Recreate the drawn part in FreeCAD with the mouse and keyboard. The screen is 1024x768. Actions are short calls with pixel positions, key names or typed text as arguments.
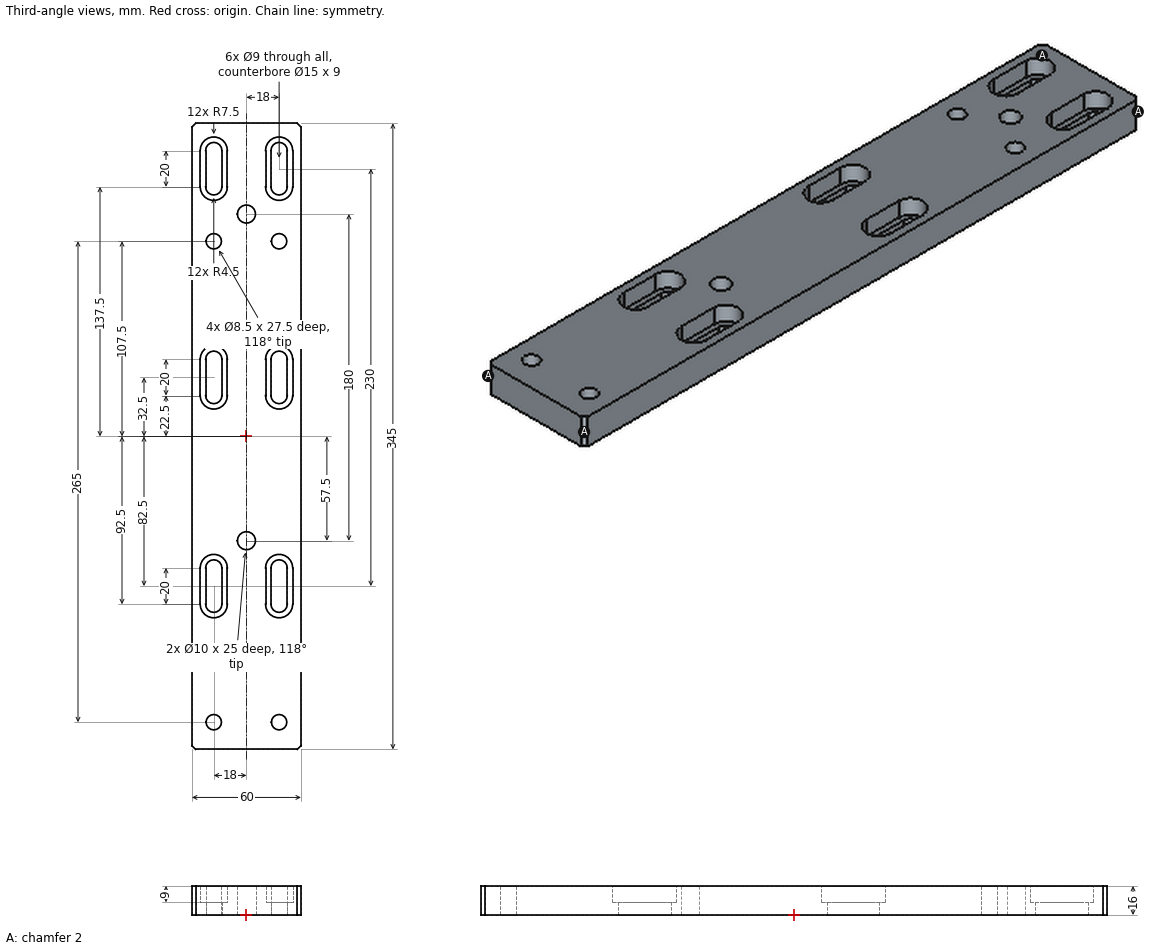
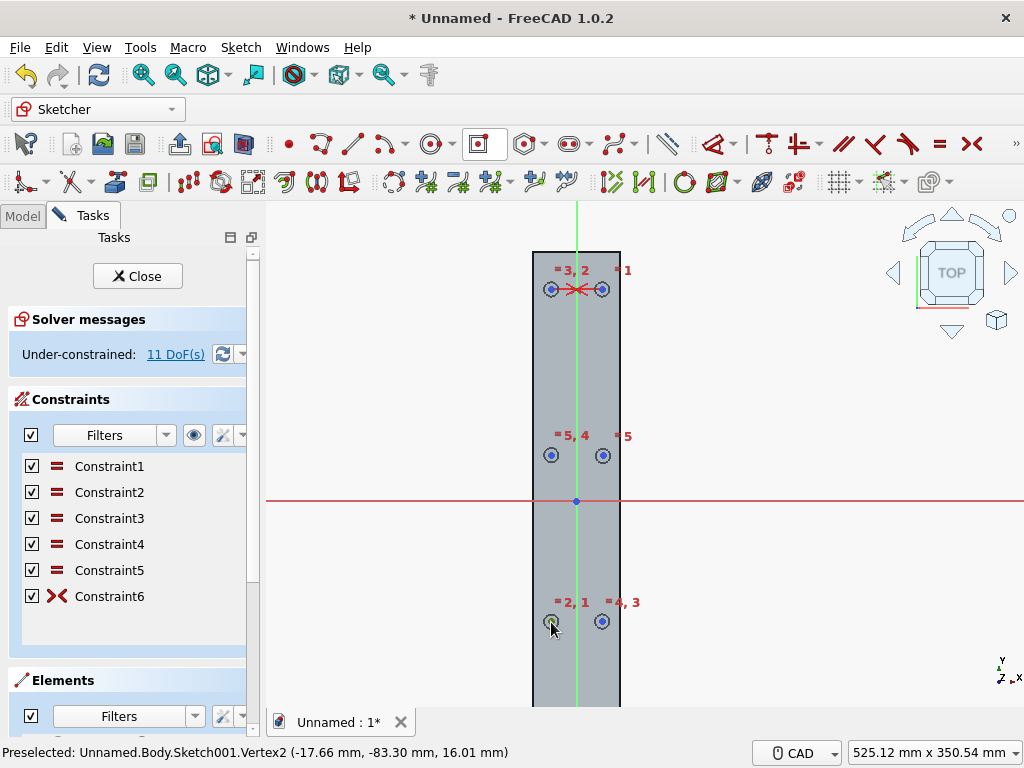
click(602, 622)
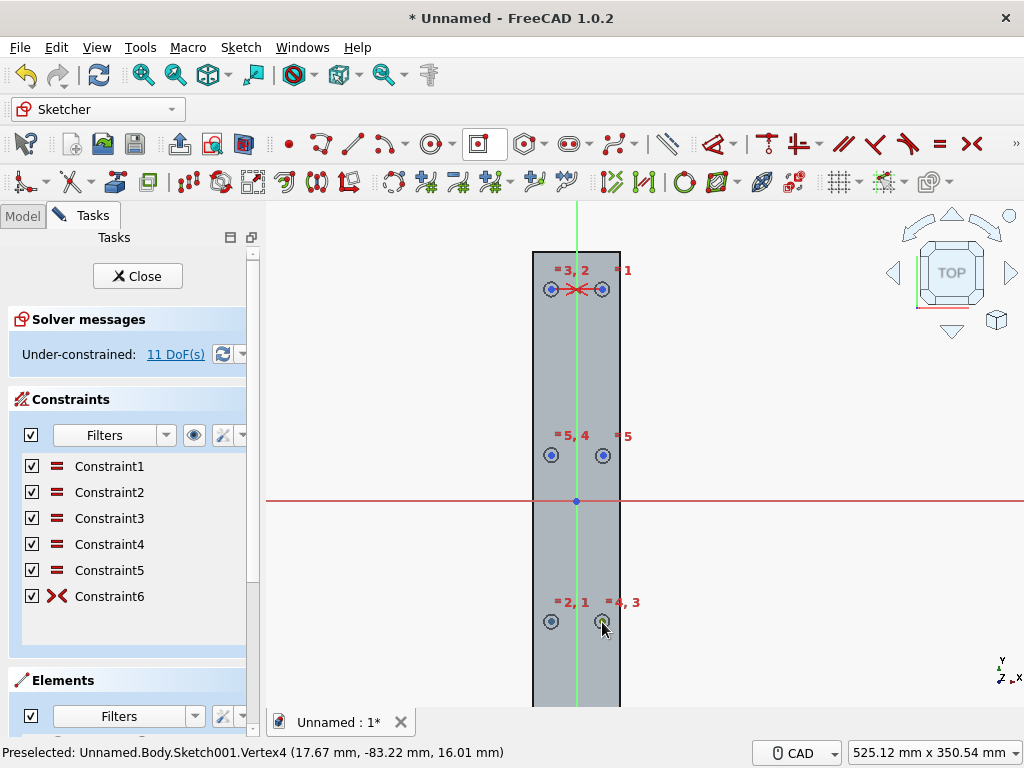
click(577, 583)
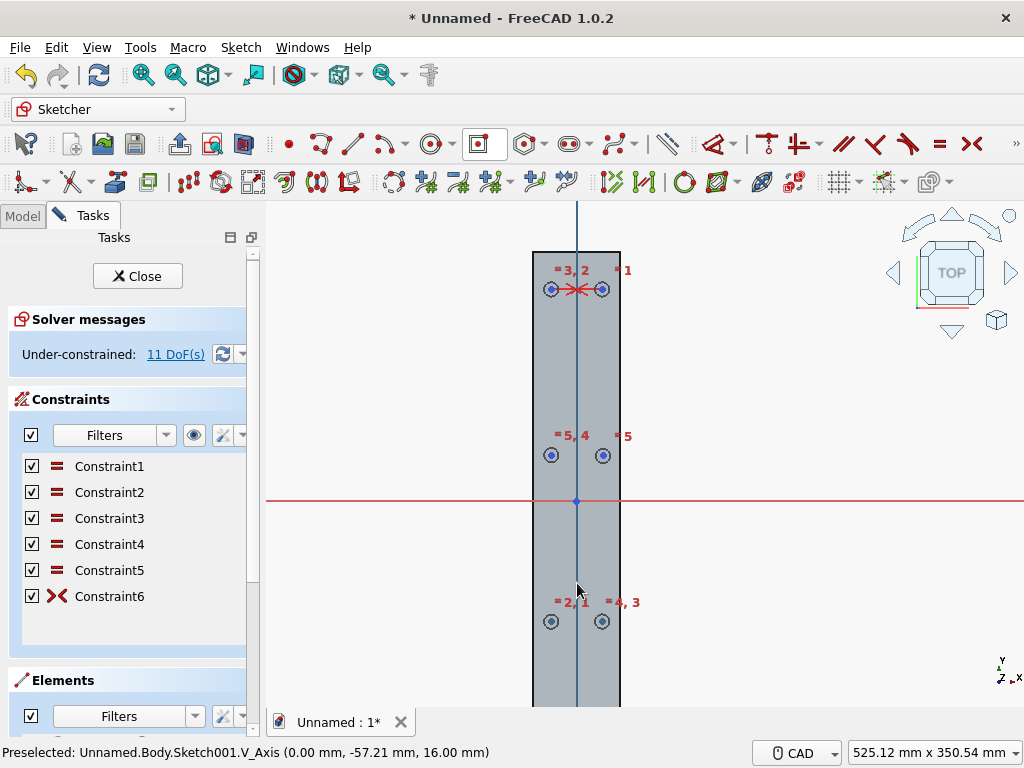
click(972, 144)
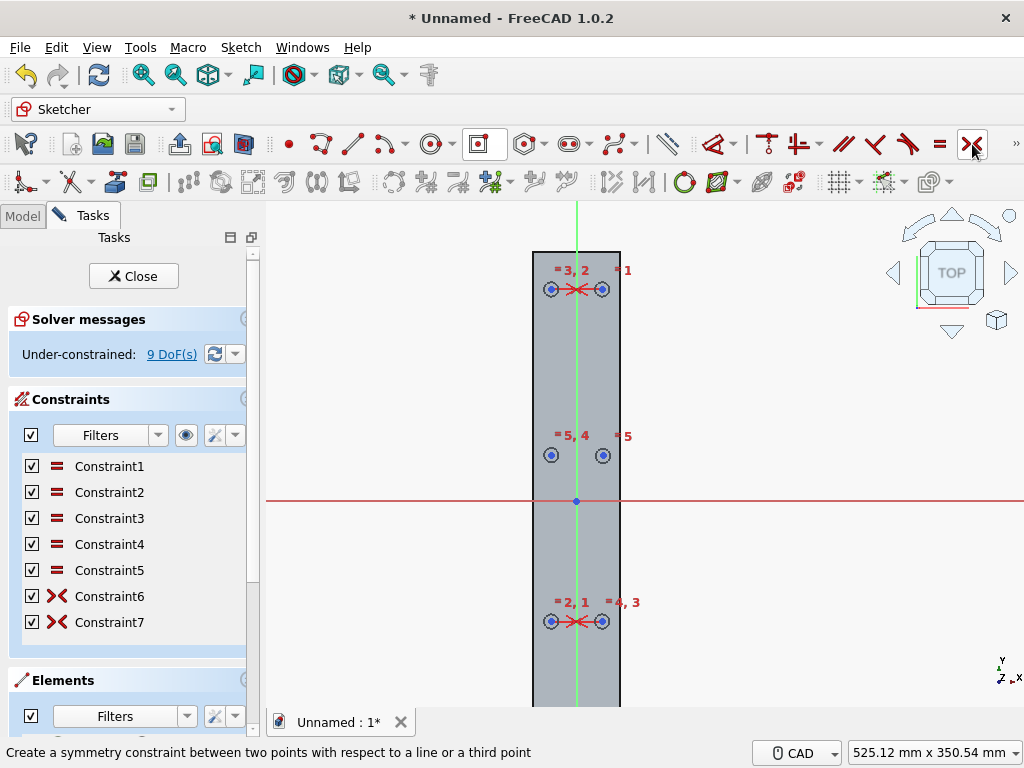
click(551, 455)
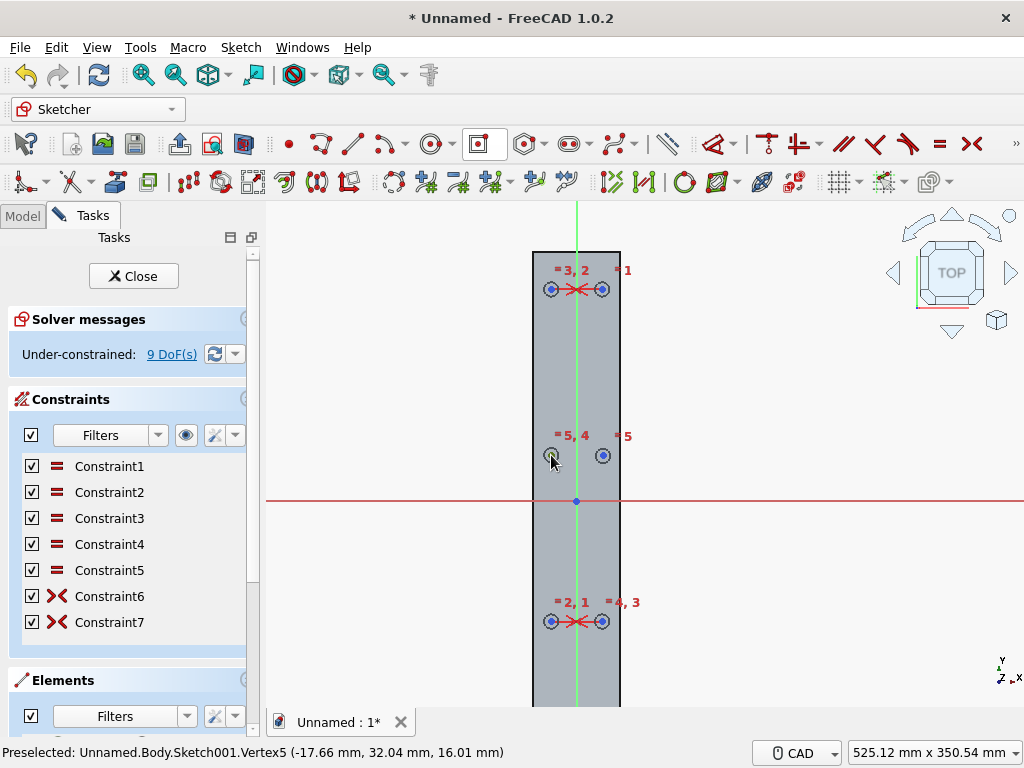
click(603, 456)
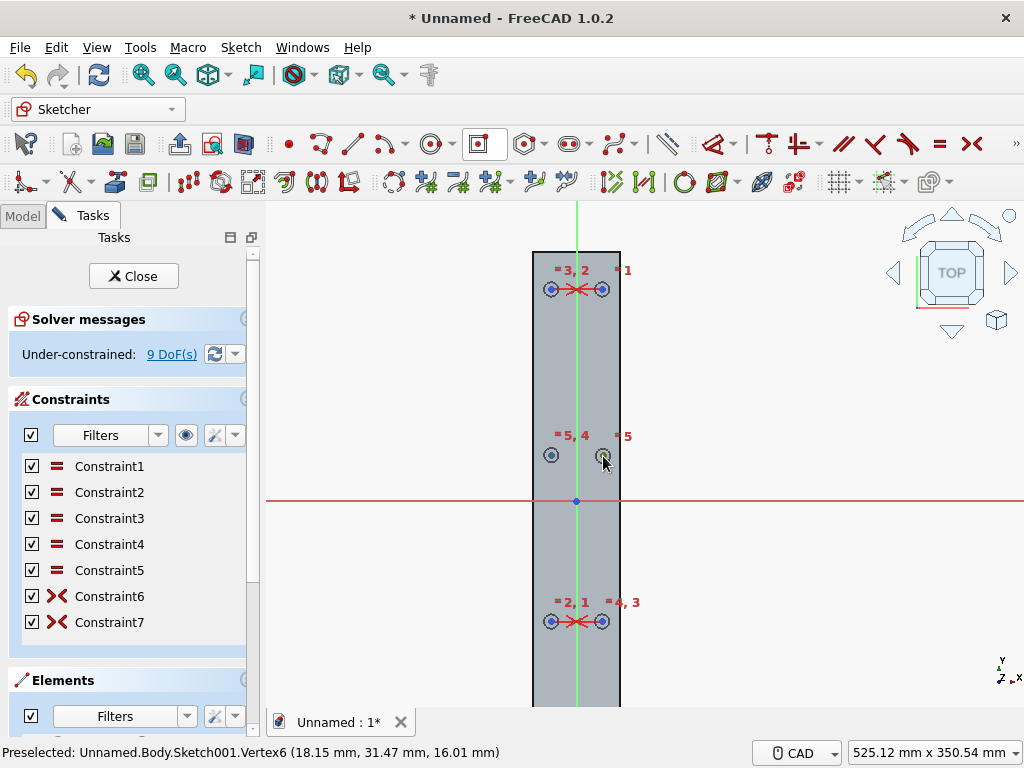
click(577, 583)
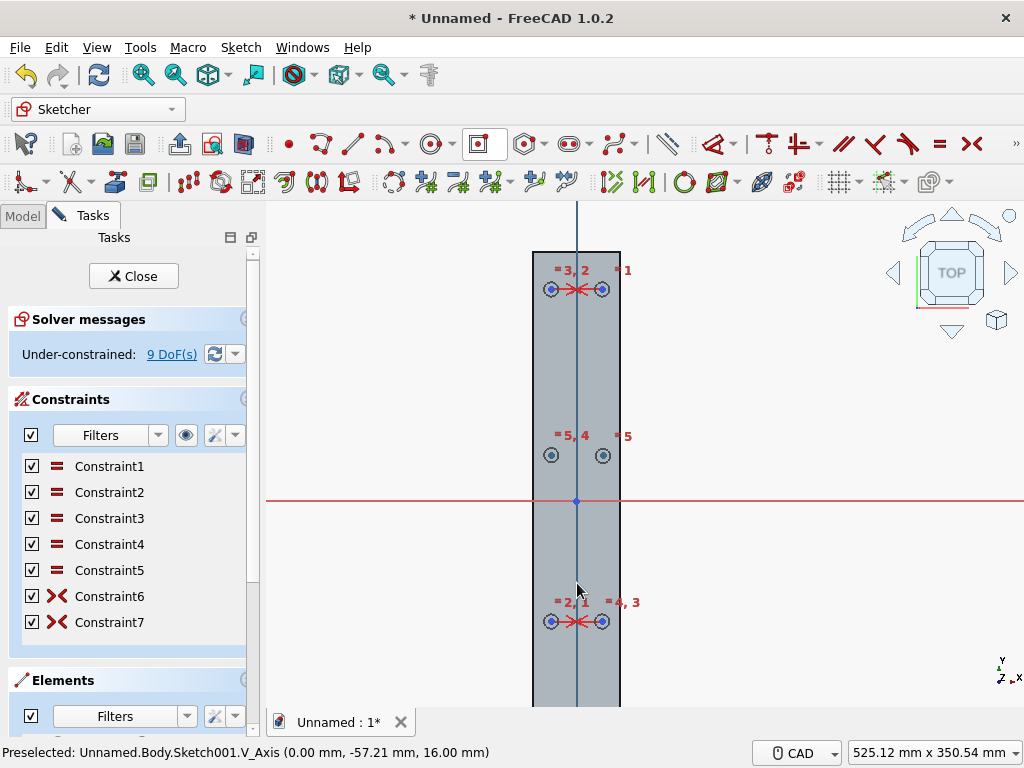
key(s)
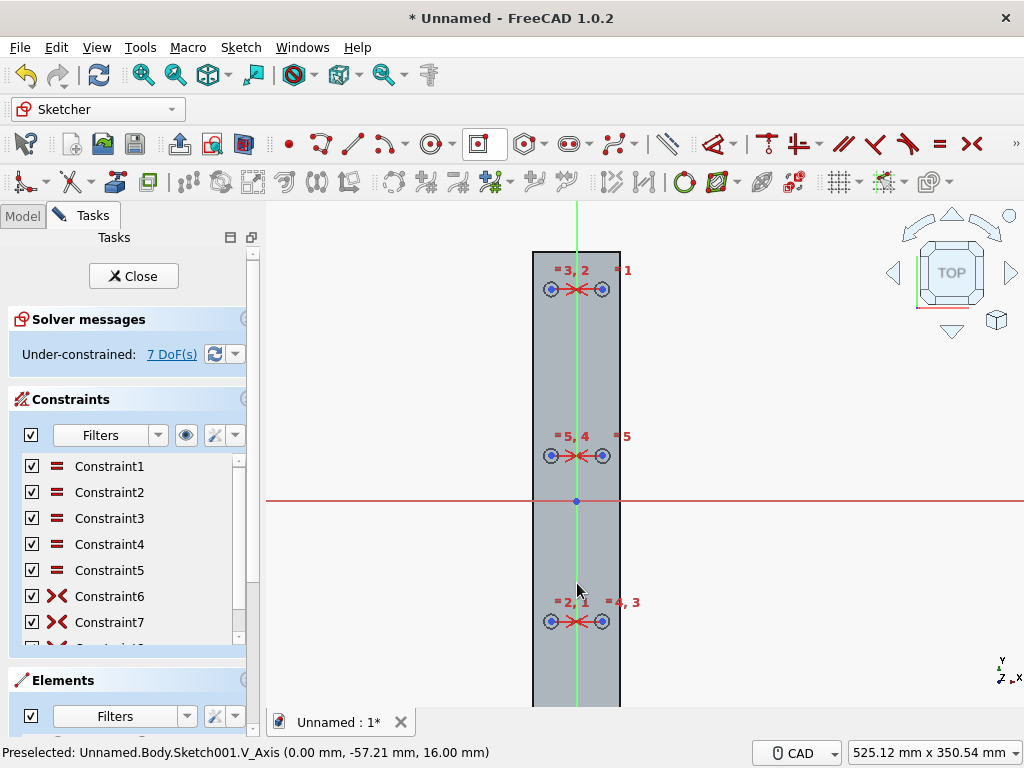
key(d)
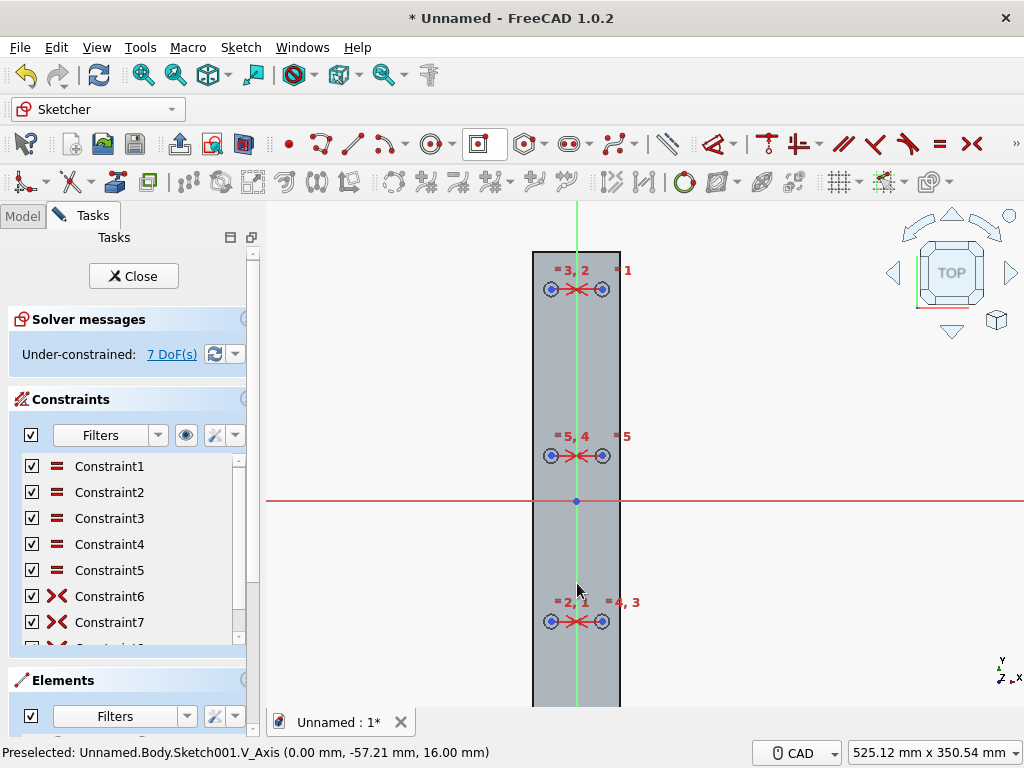
scroll(602, 282, up, 6)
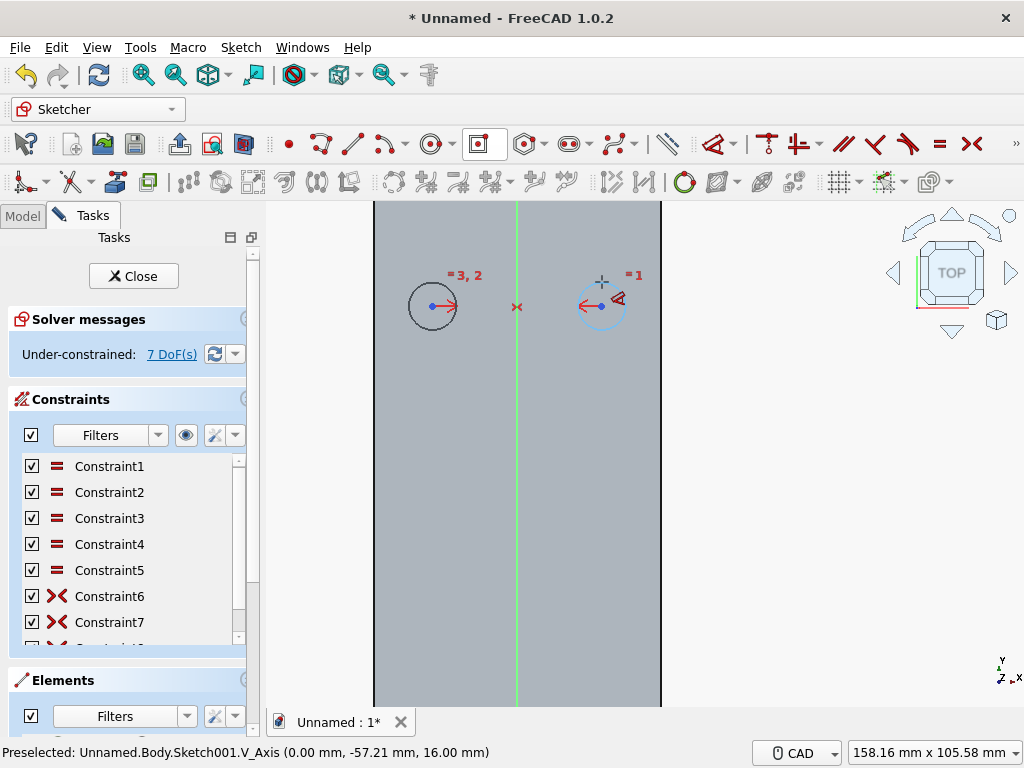
click(603, 283)
click(604, 251)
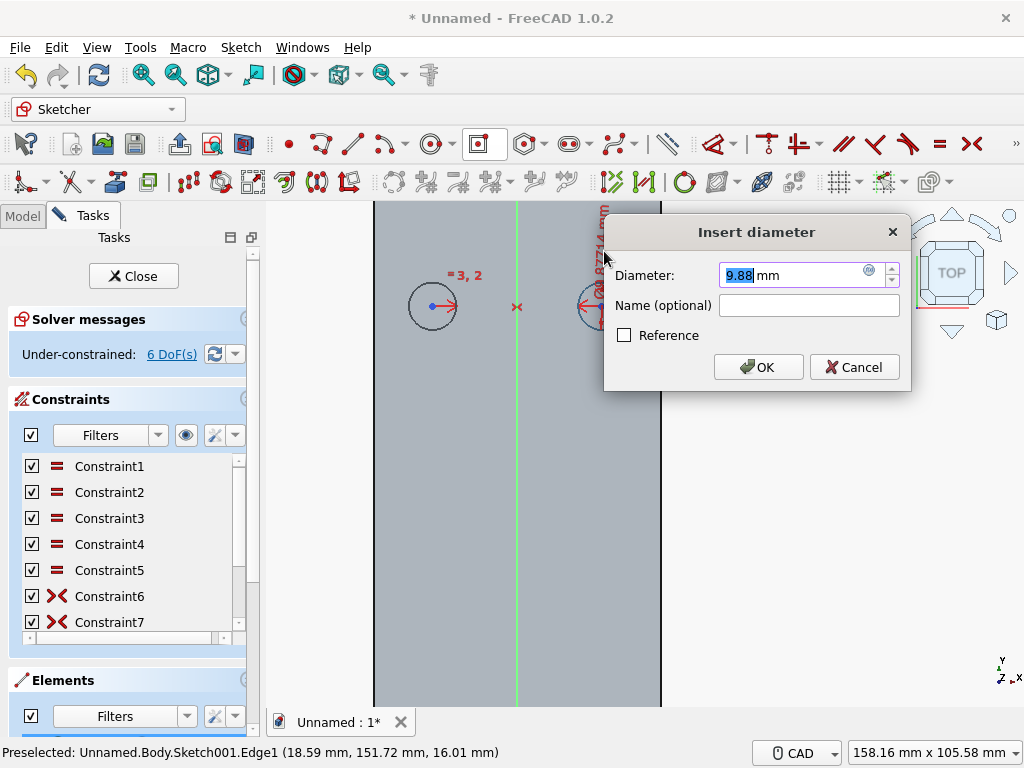
text(9)
key(Return)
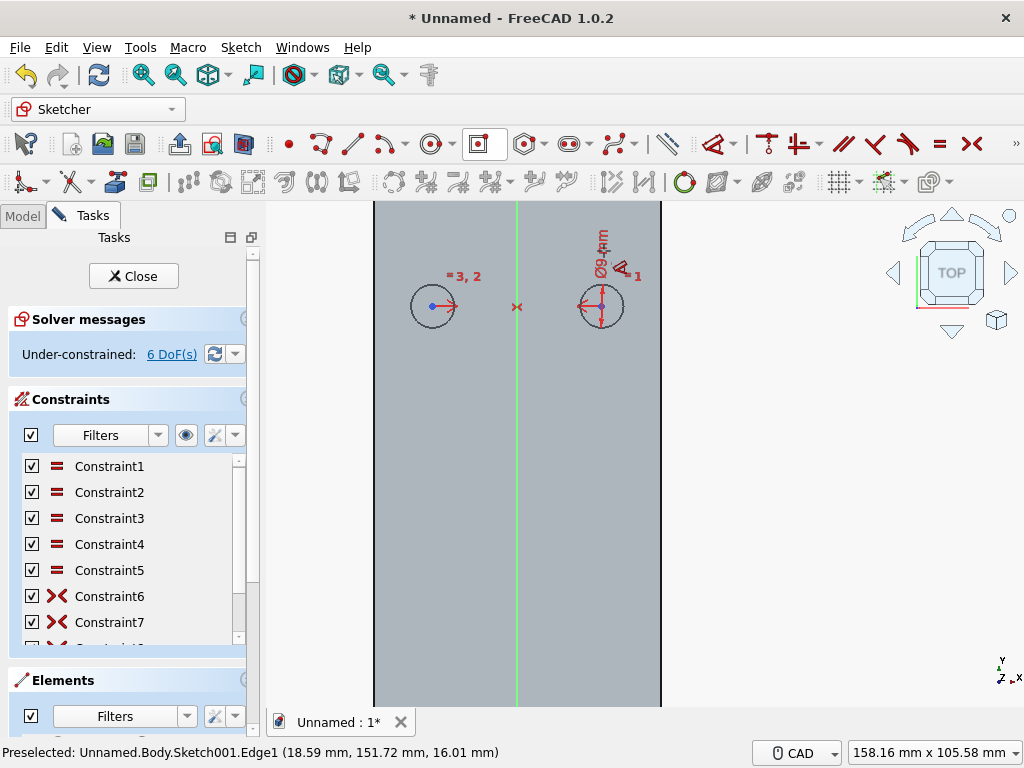
click(602, 306)
click(560, 272)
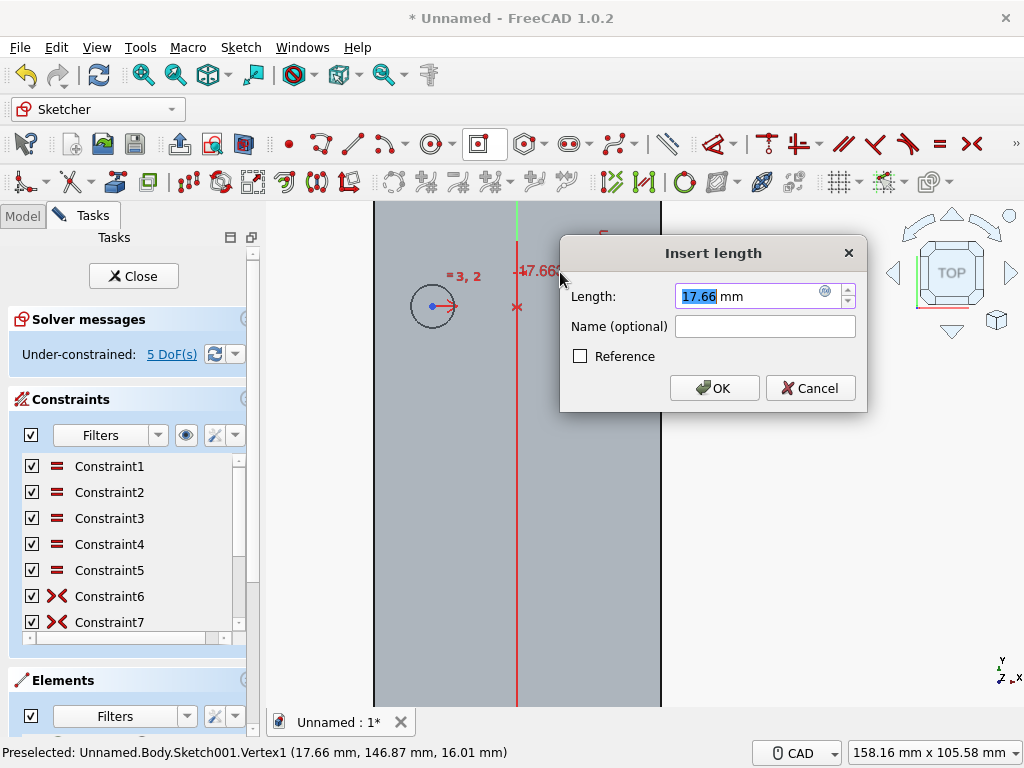
text(18)
key(Return)